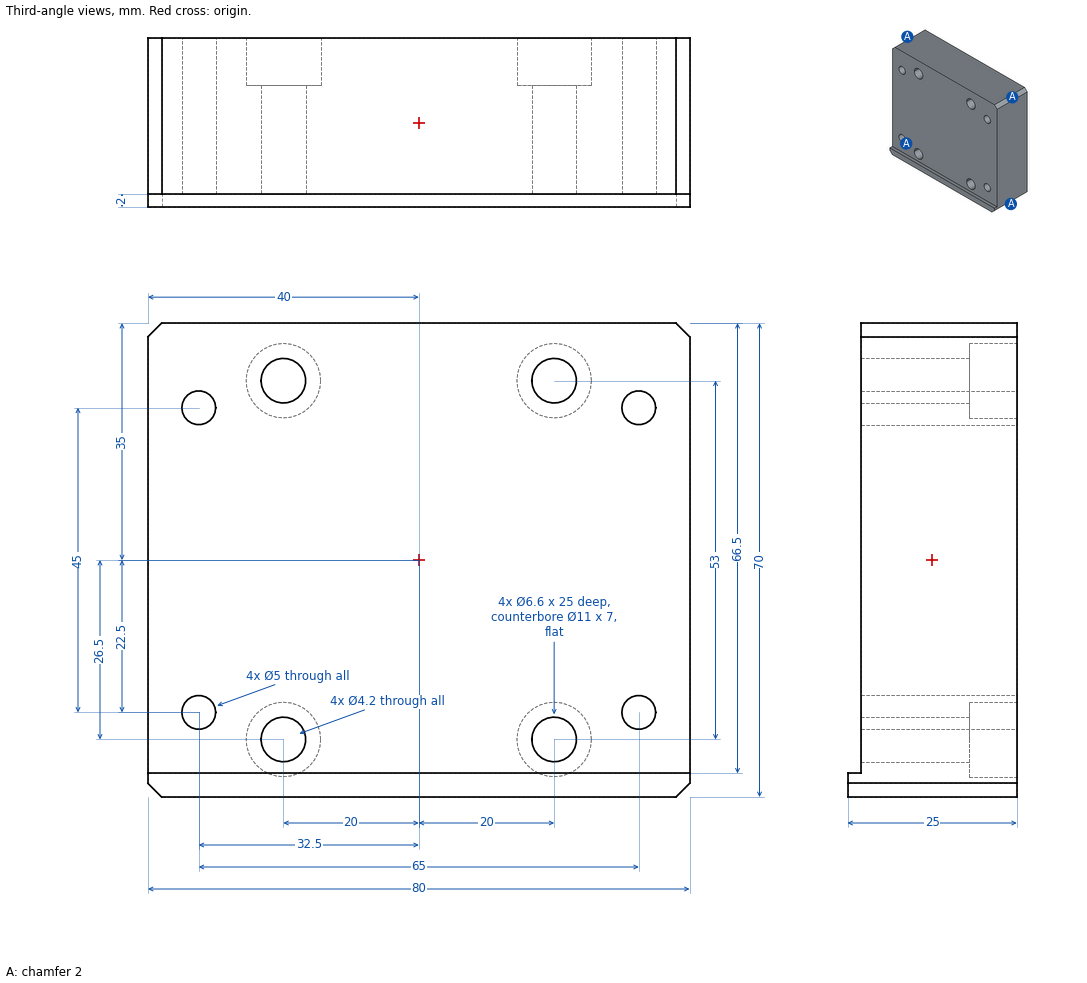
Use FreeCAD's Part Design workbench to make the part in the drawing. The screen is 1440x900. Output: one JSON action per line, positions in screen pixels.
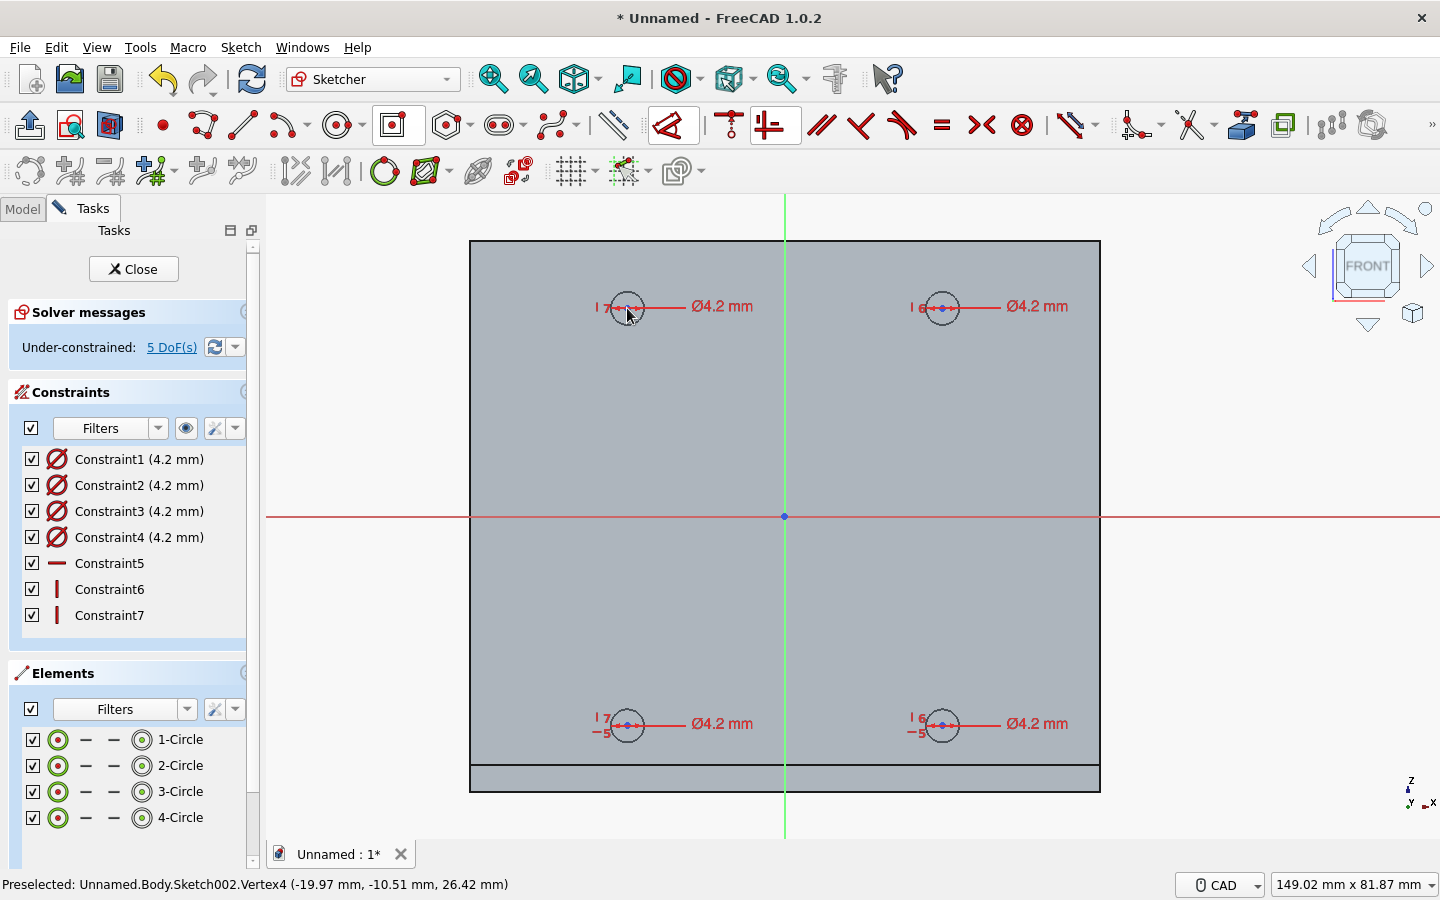
{"action": "left_click", "coordinate": [943, 308]}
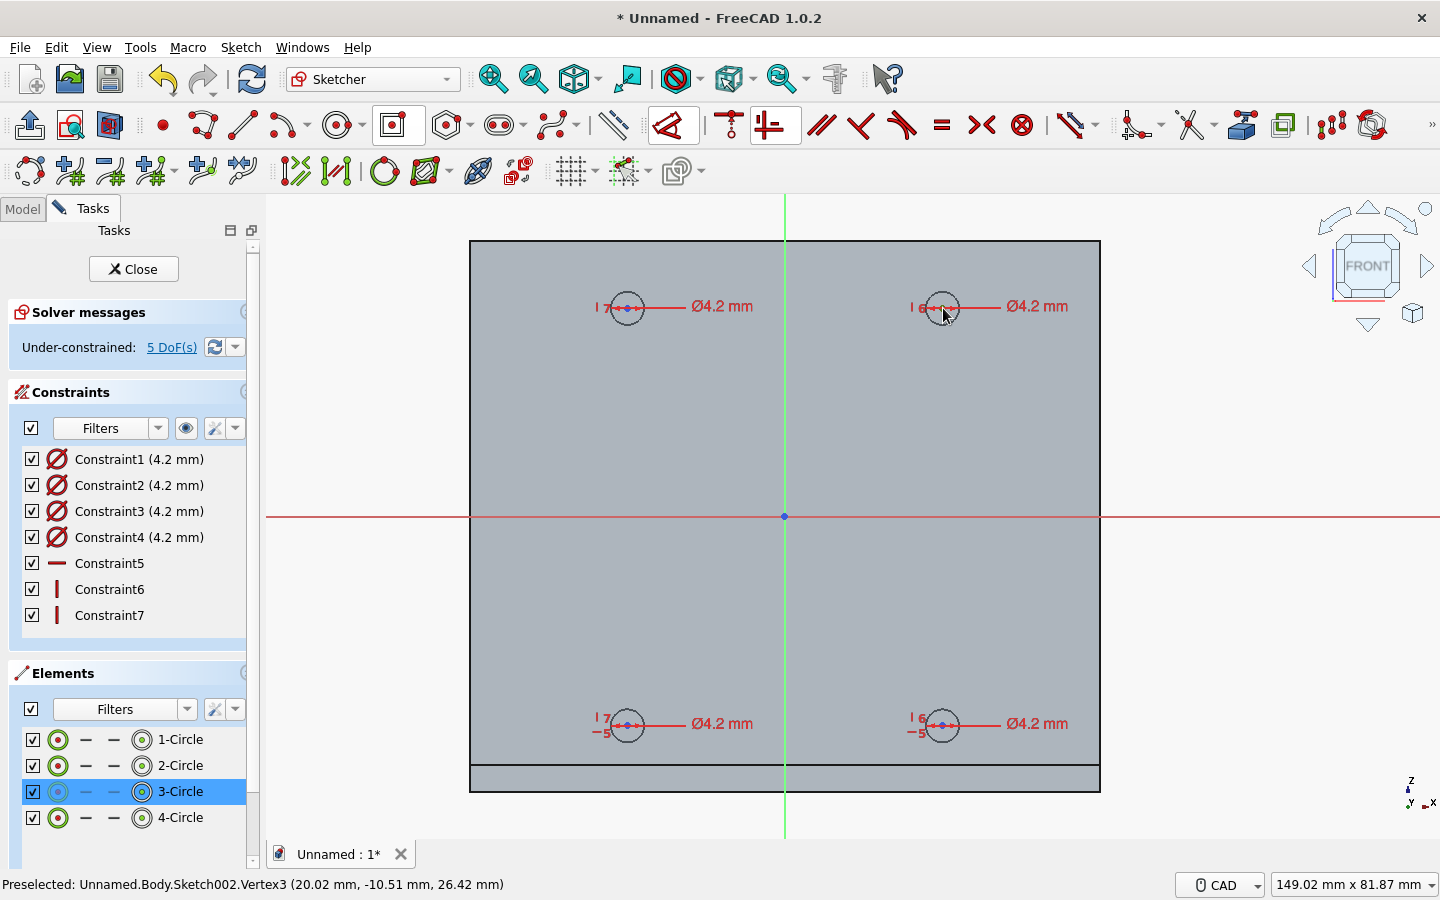
{"action": "left_click", "coordinate": [627, 308]}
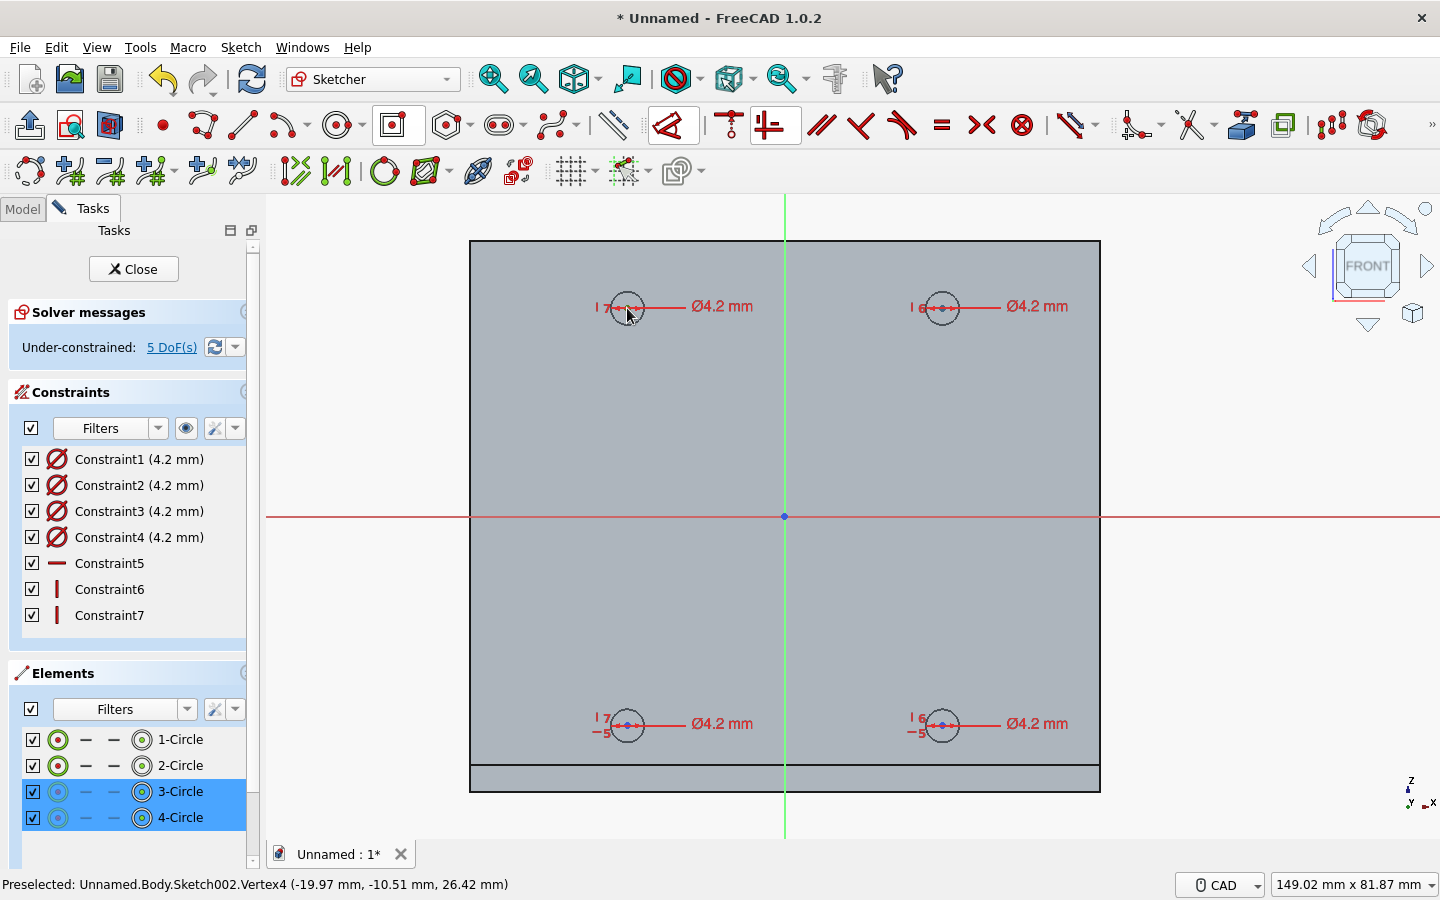
{"action": "left_click", "coordinate": [796, 126]}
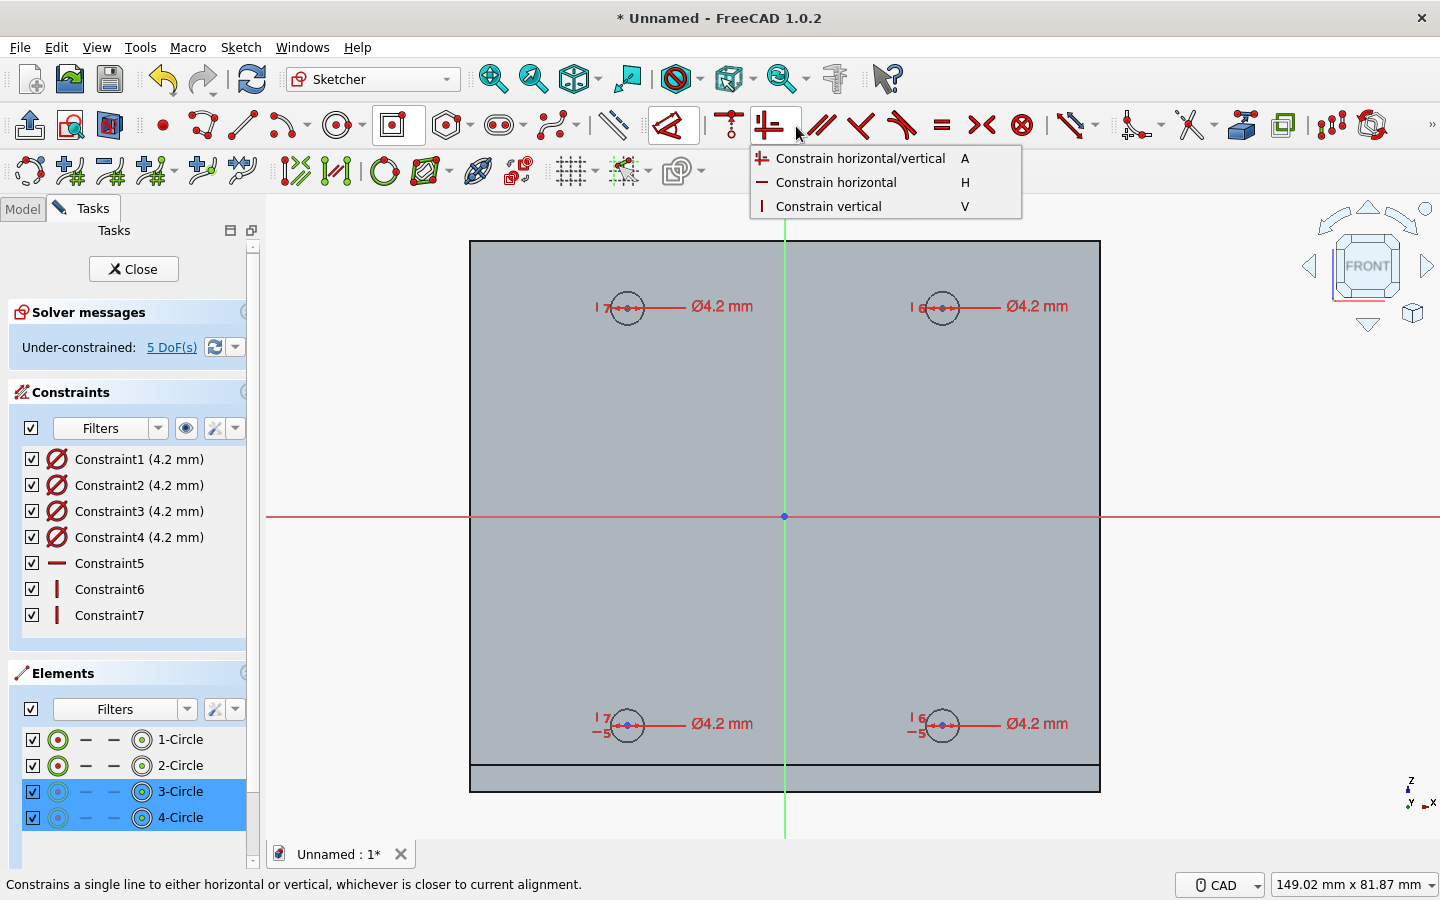
{"action": "left_click", "coordinate": [886, 182]}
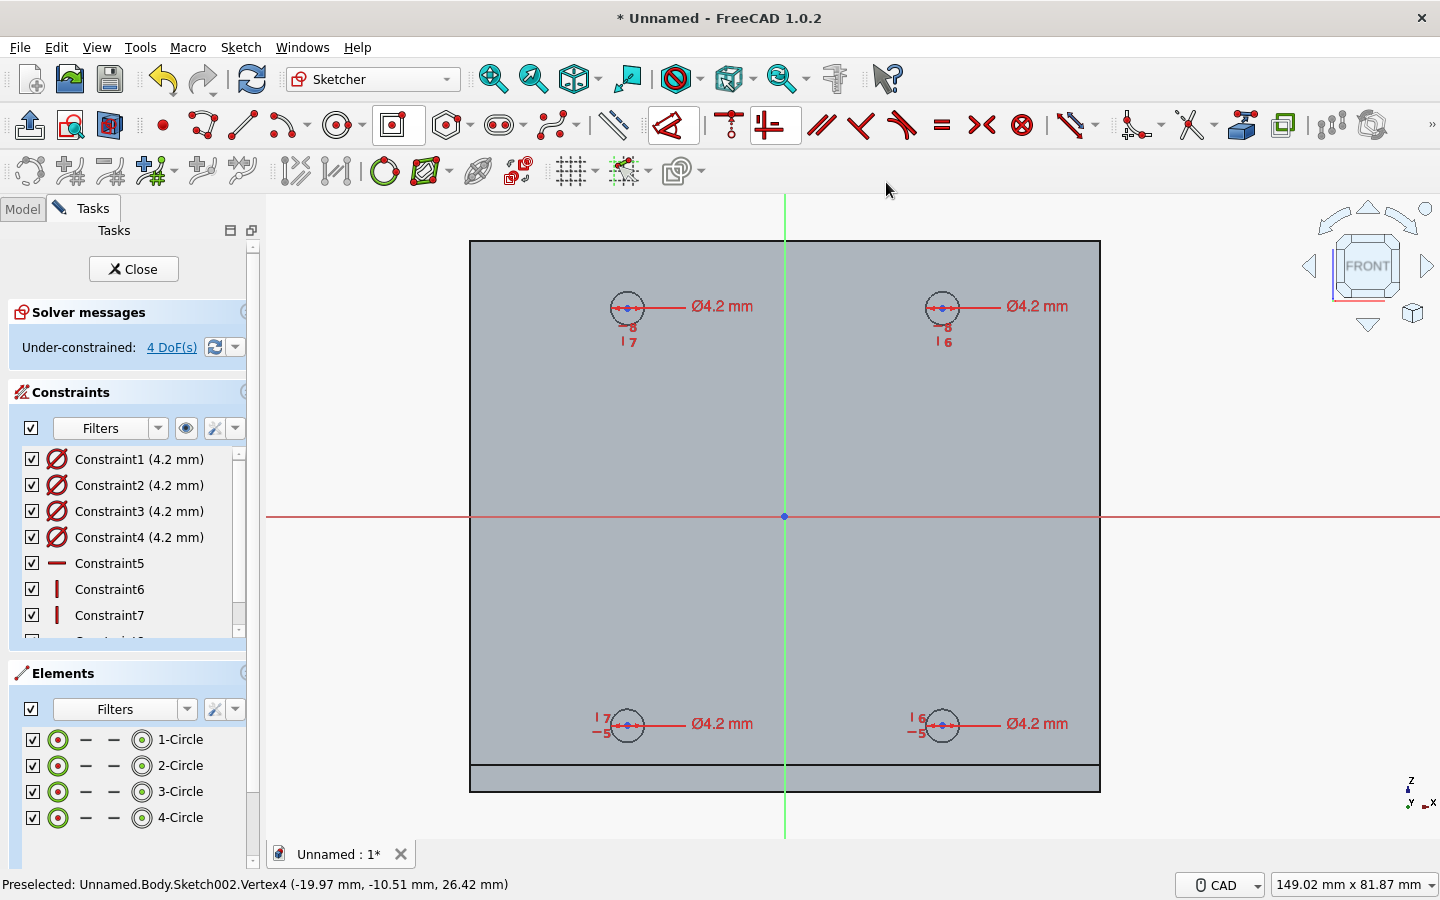
{"action": "left_click", "coordinate": [627, 726]}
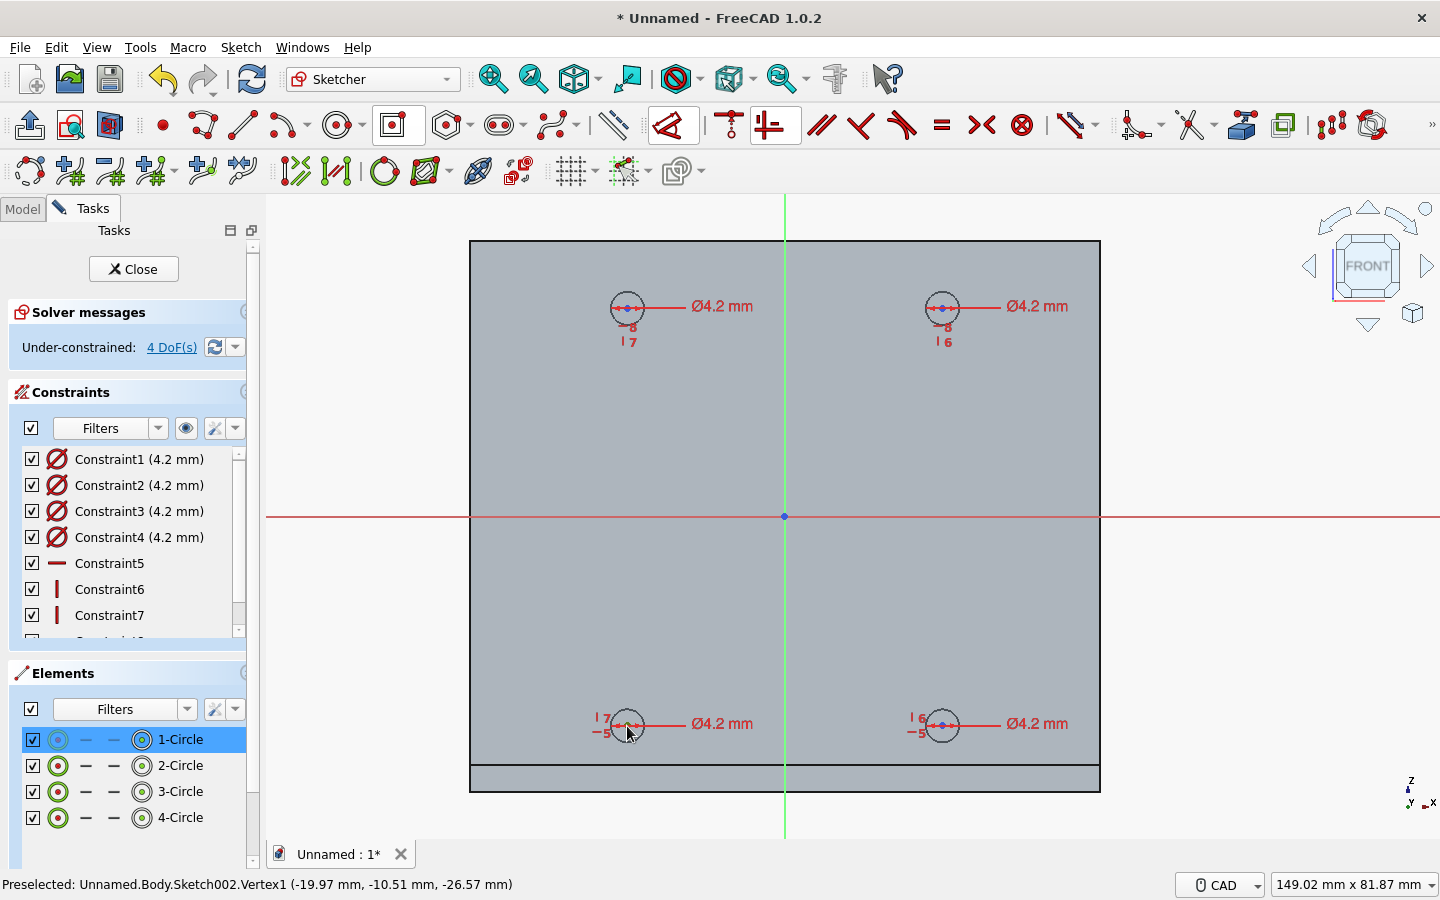
{"action": "left_click", "coordinate": [694, 126]}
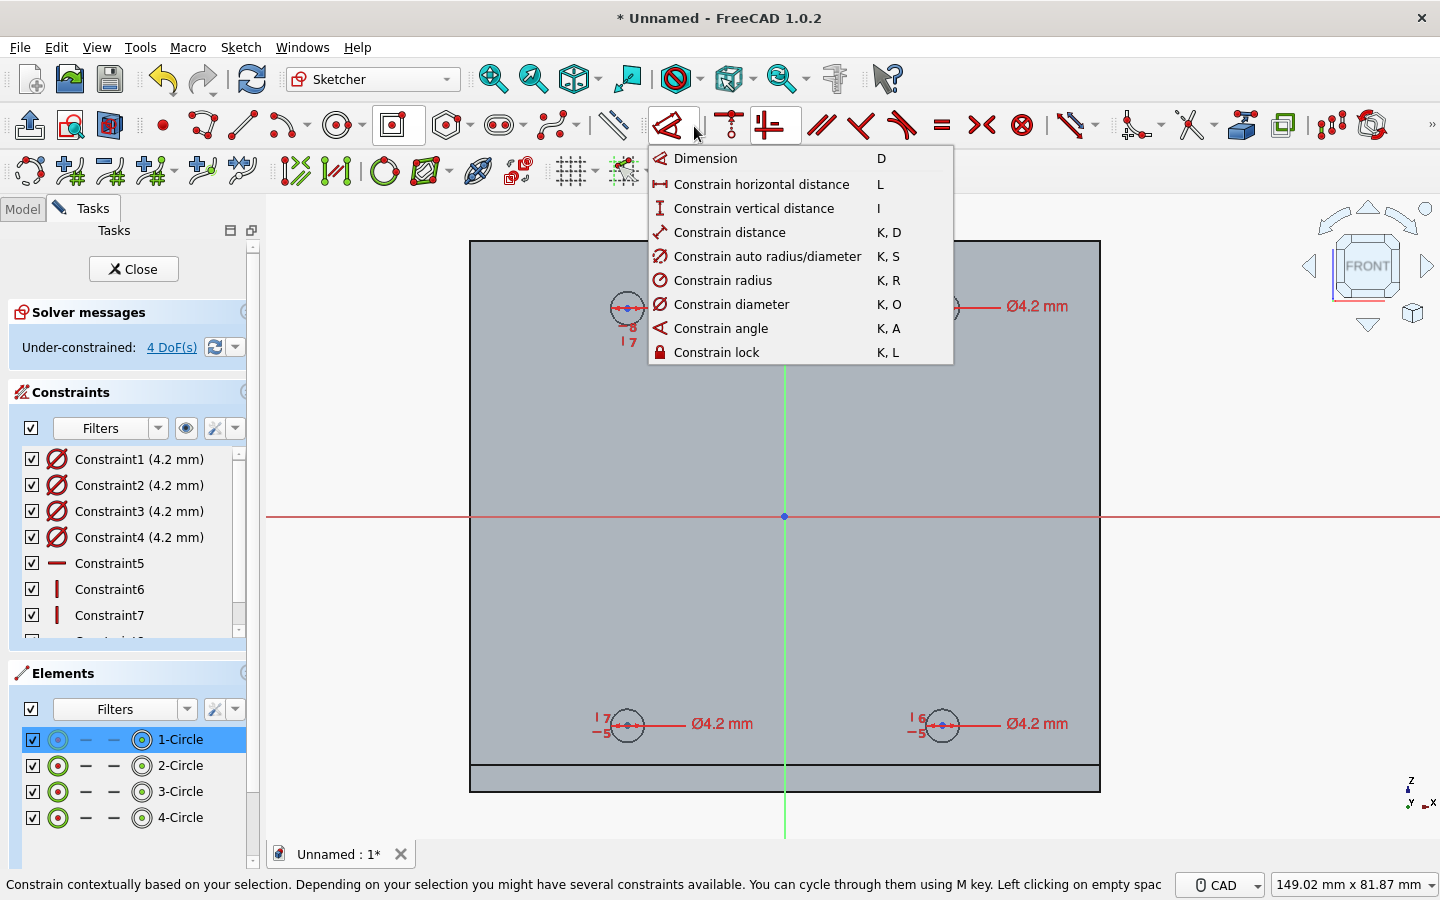
{"action": "left_click", "coordinate": [801, 184]}